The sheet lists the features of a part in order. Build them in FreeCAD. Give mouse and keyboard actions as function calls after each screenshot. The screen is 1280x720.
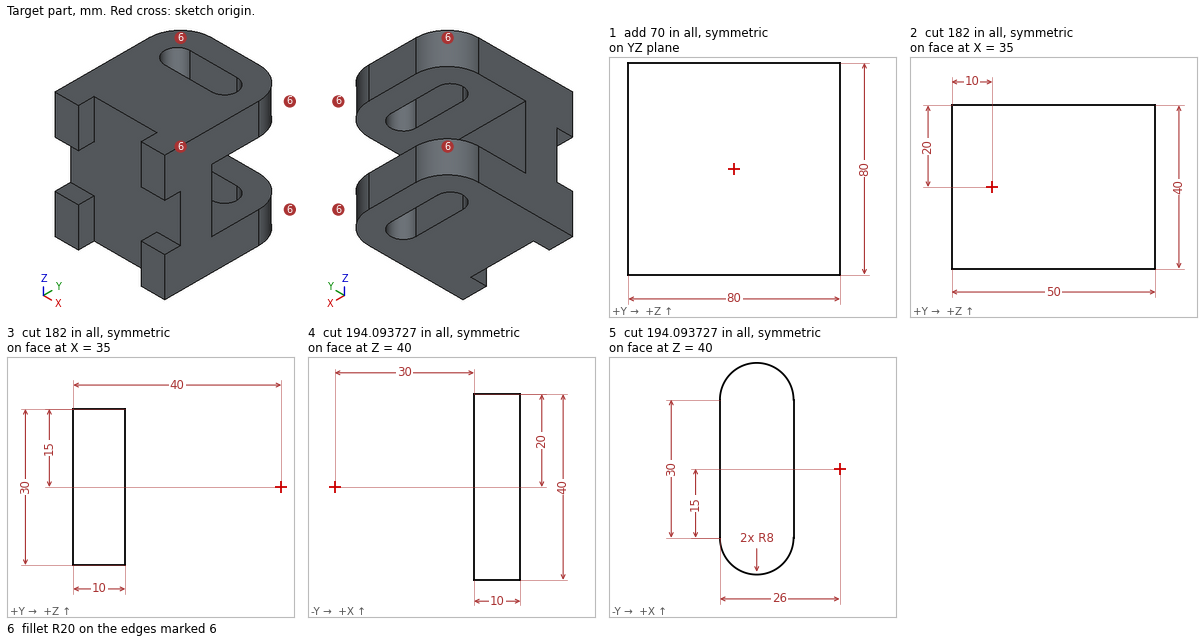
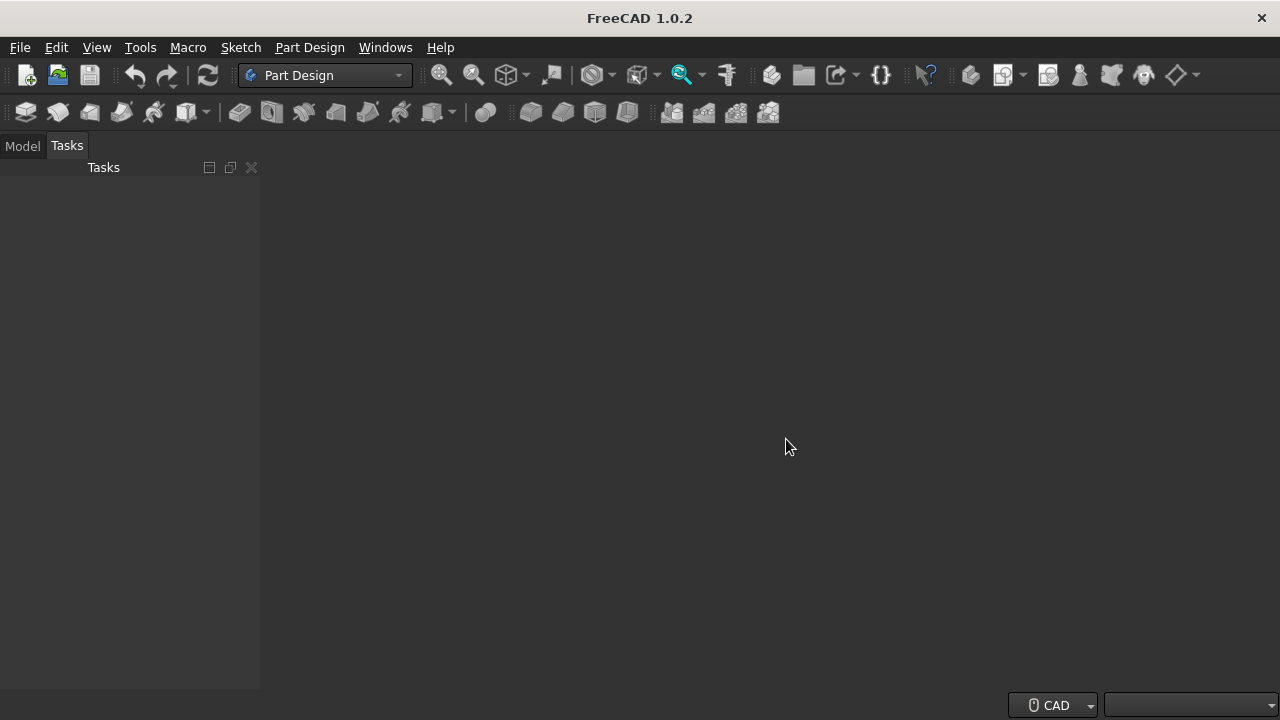
key(ctrl+n)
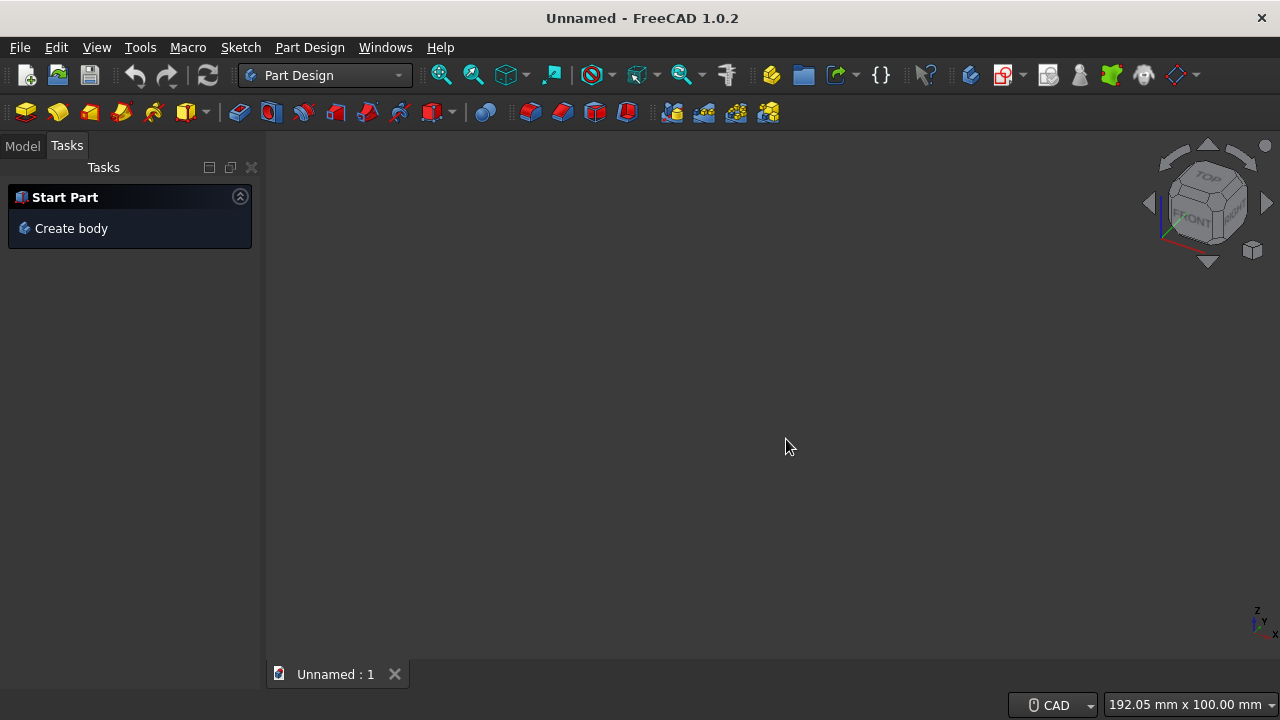
click(1004, 76)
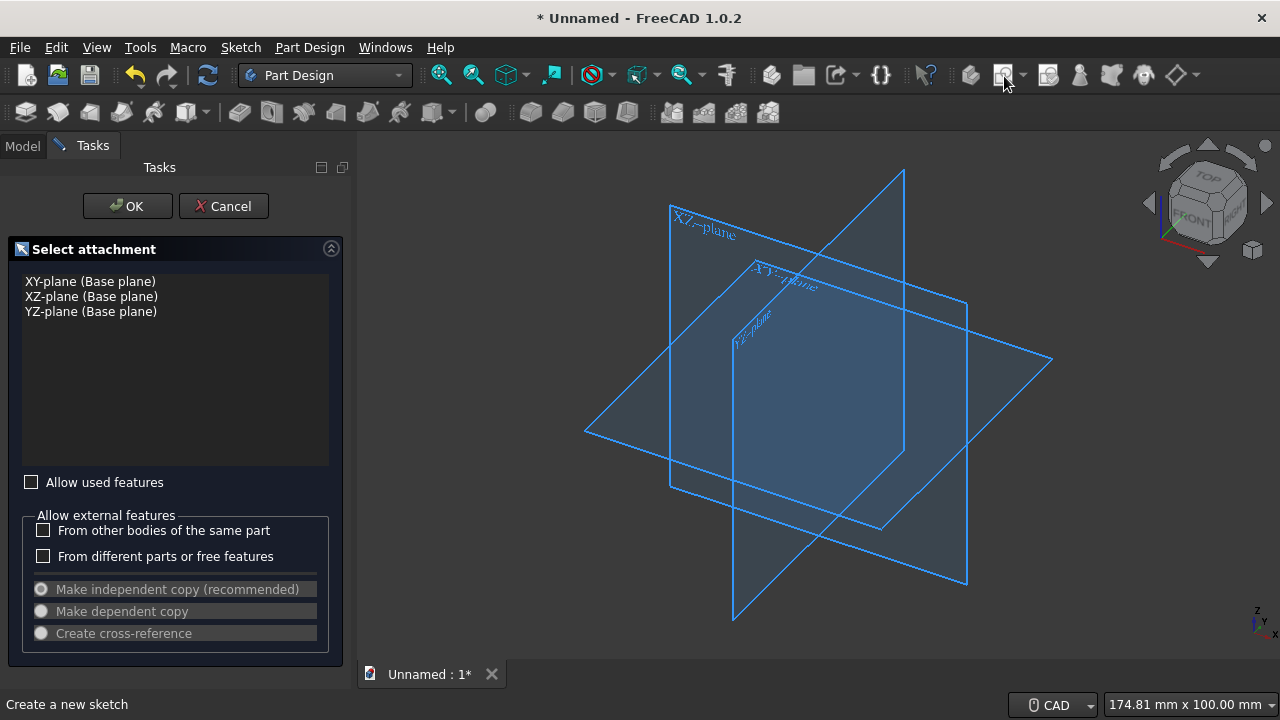
click(82, 312)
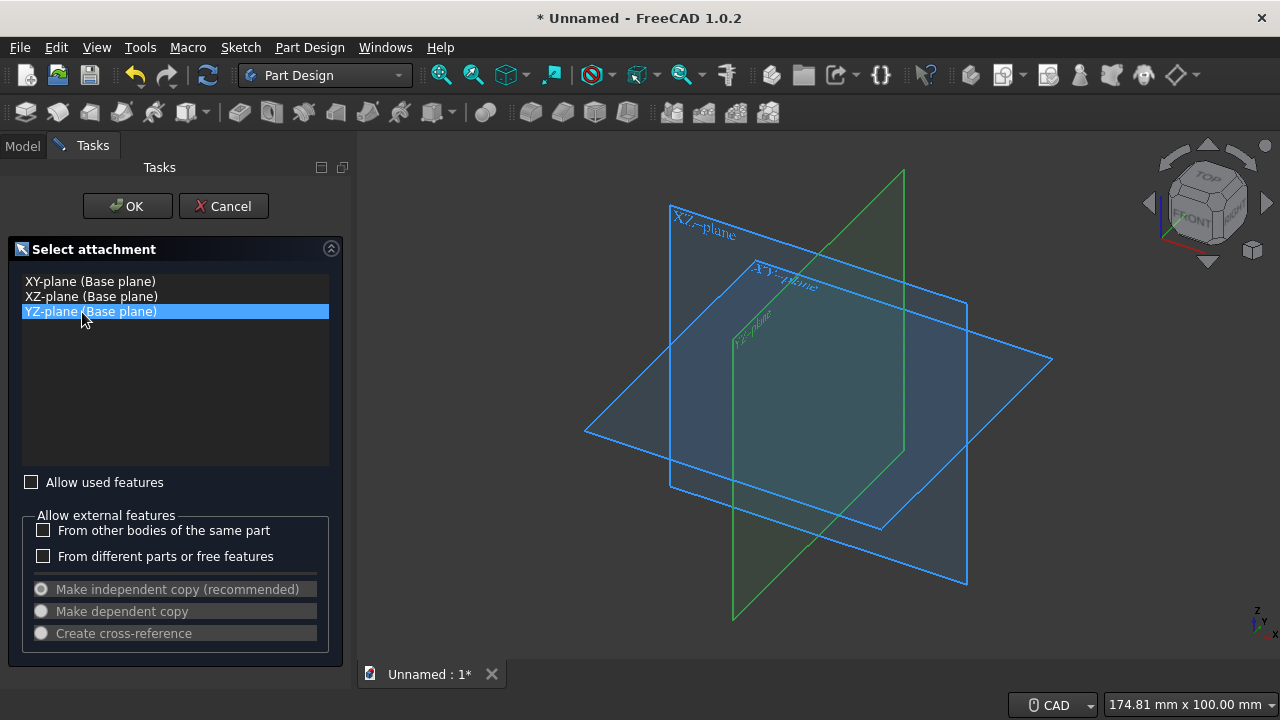
click(128, 206)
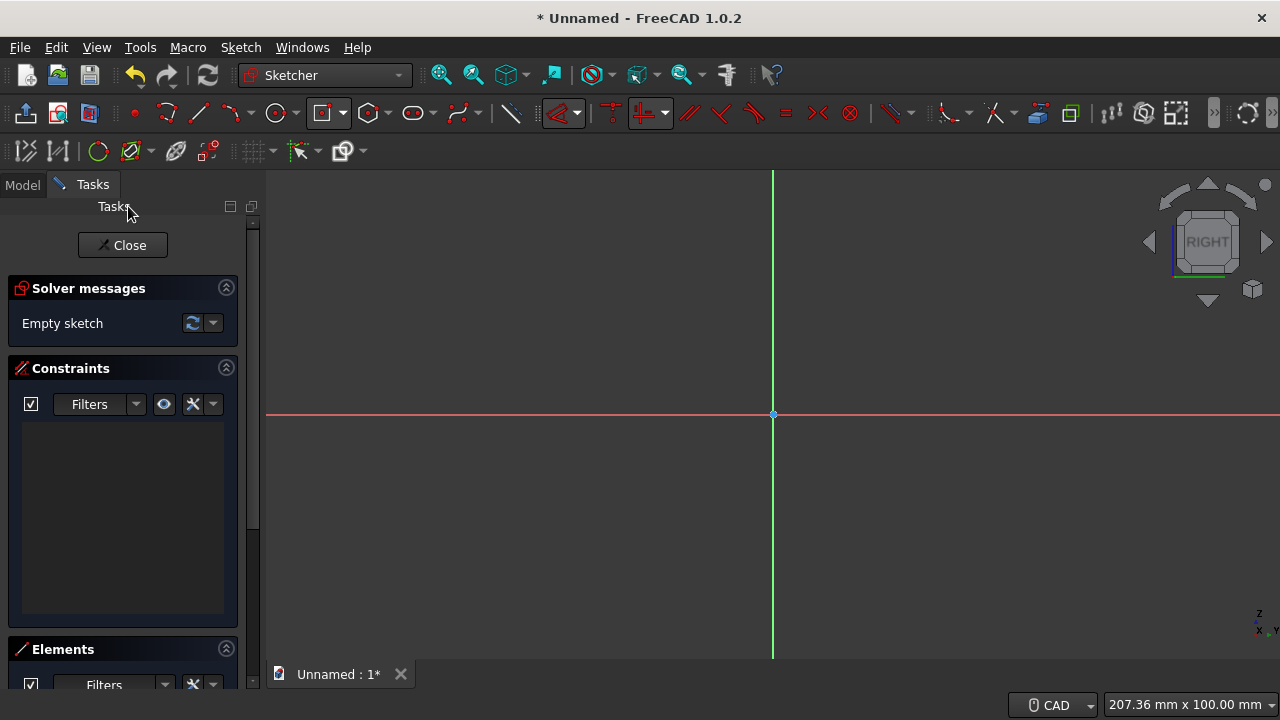
scroll(395, 415, down, 1)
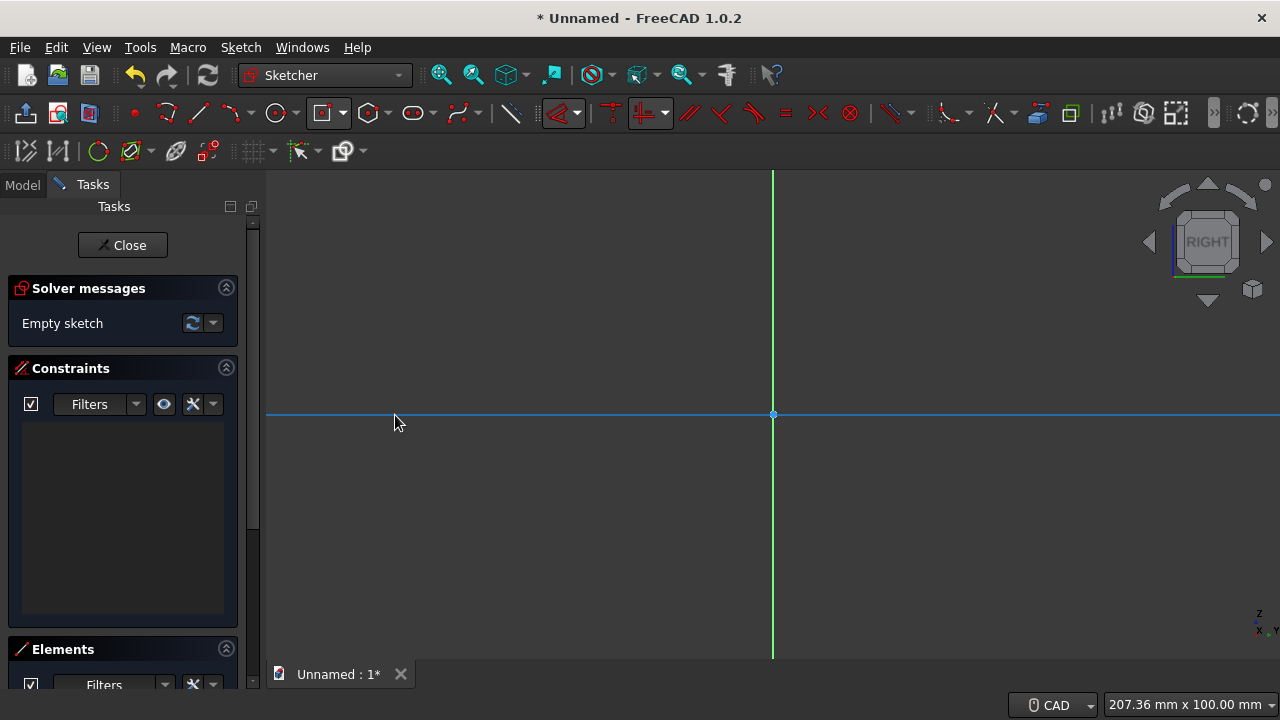
key(g)
key(v)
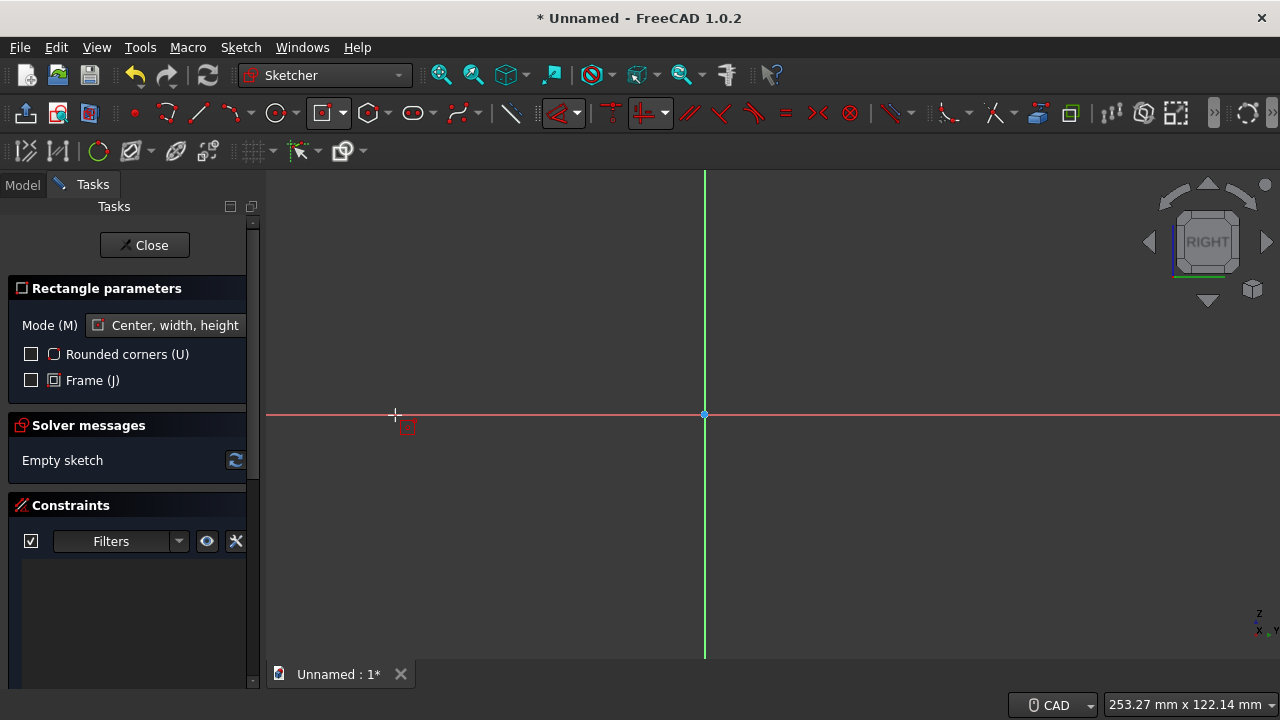
click(705, 415)
move(865, 255)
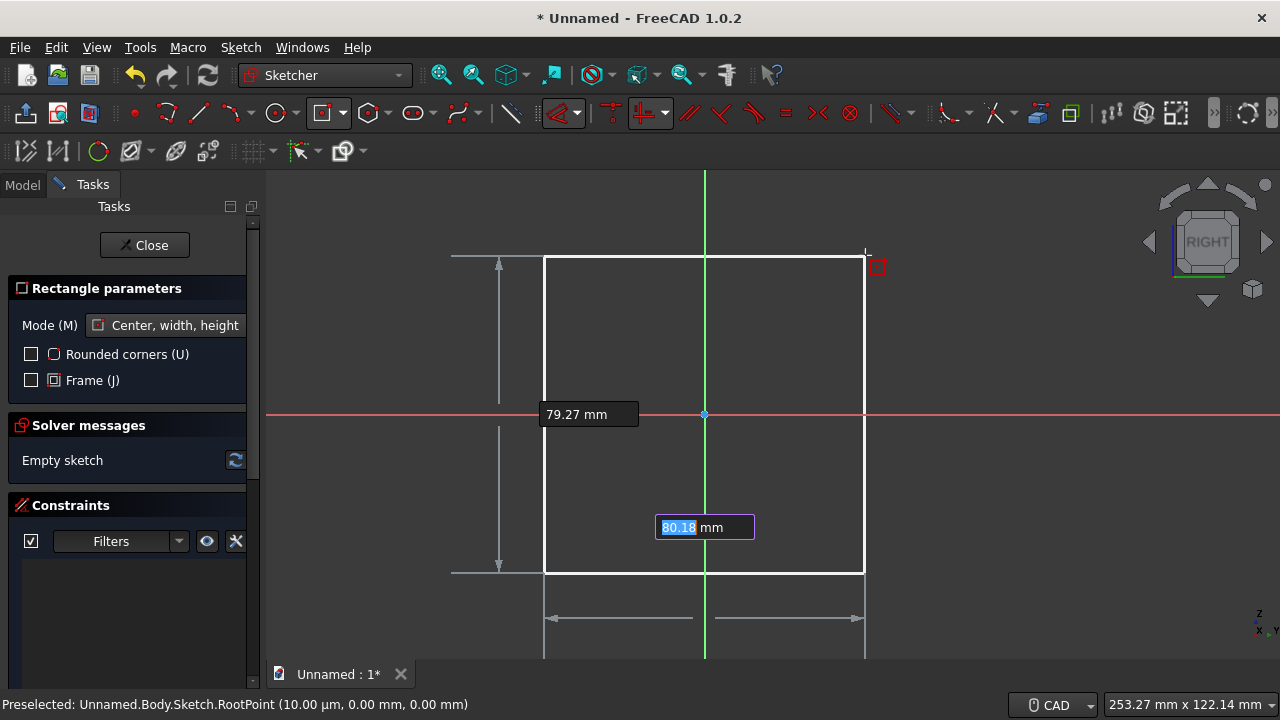
text(80)
key(Tab)
text(80)
key(Return)
key(Escape)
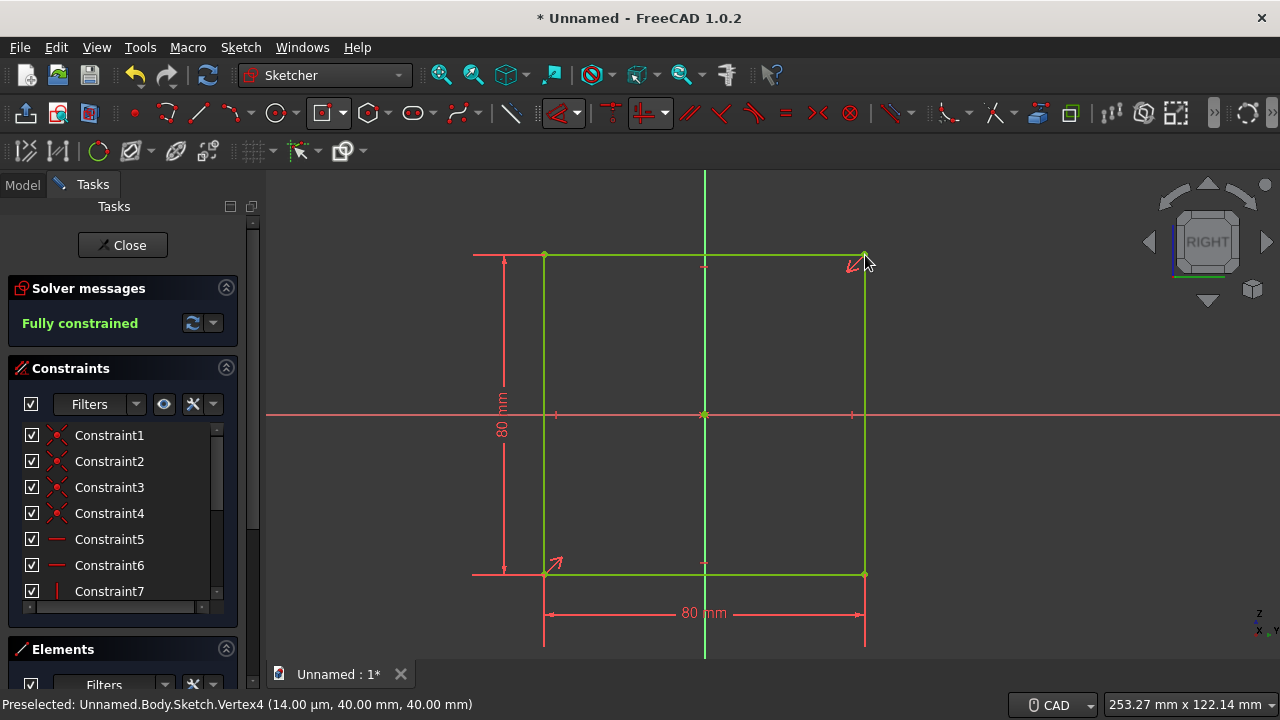
click(123, 245)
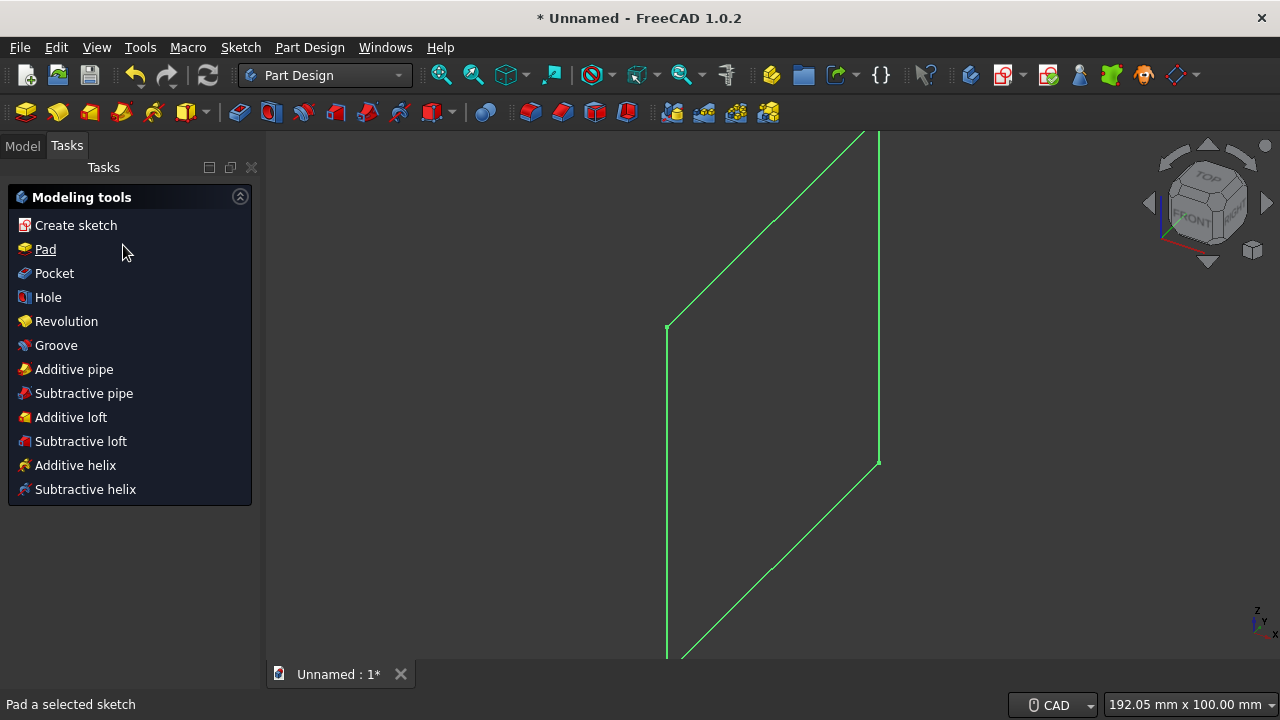
click(26, 112)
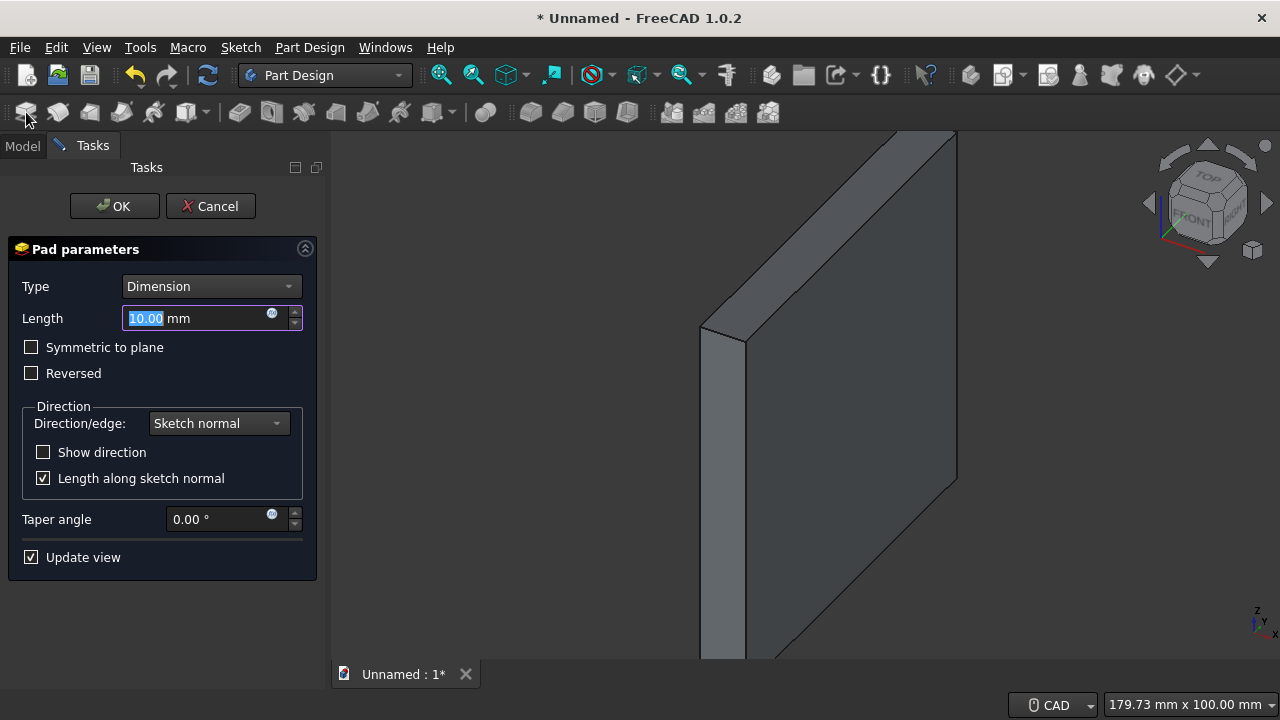
text(70)
key(Tab)